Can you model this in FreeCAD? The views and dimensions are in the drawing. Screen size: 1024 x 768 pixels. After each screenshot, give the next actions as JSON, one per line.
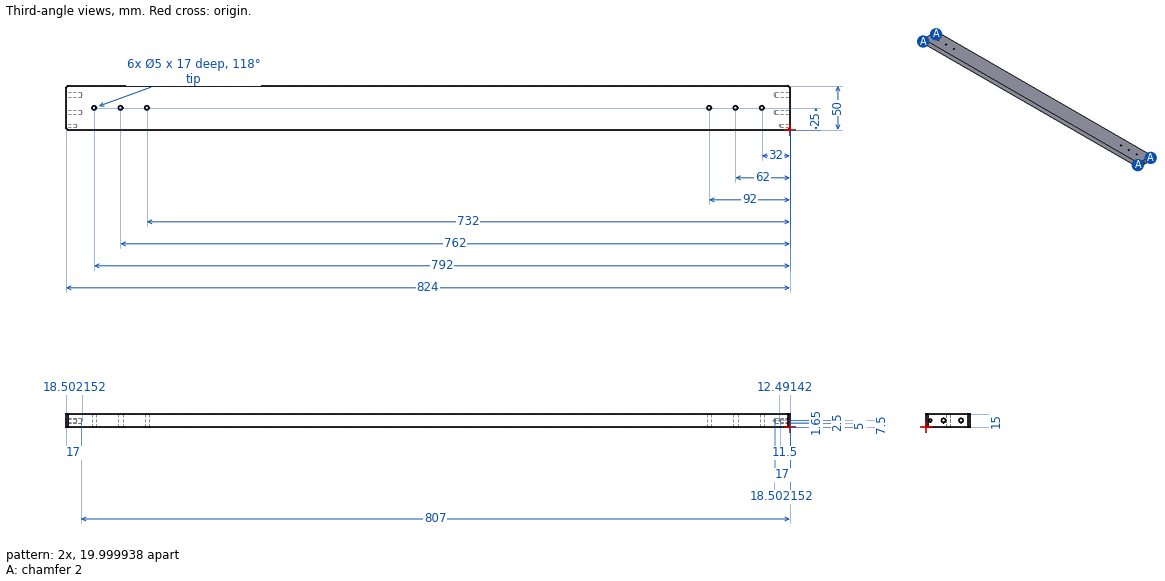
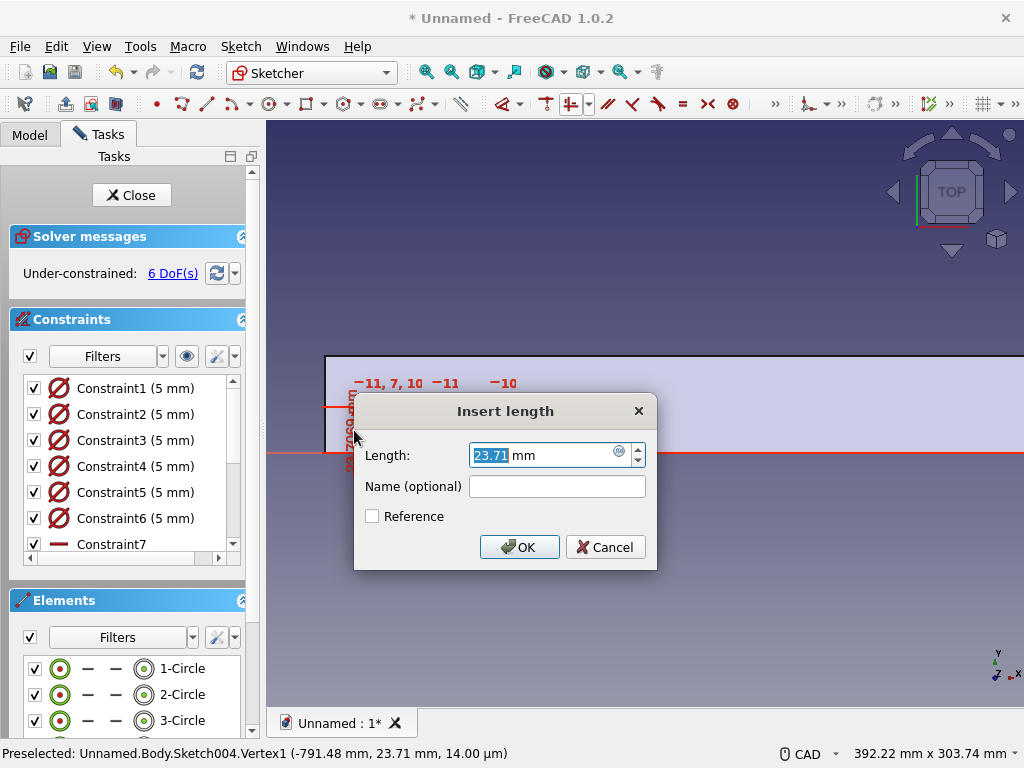
{"action": "type", "text": "25"}
{"action": "key", "text": "Return"}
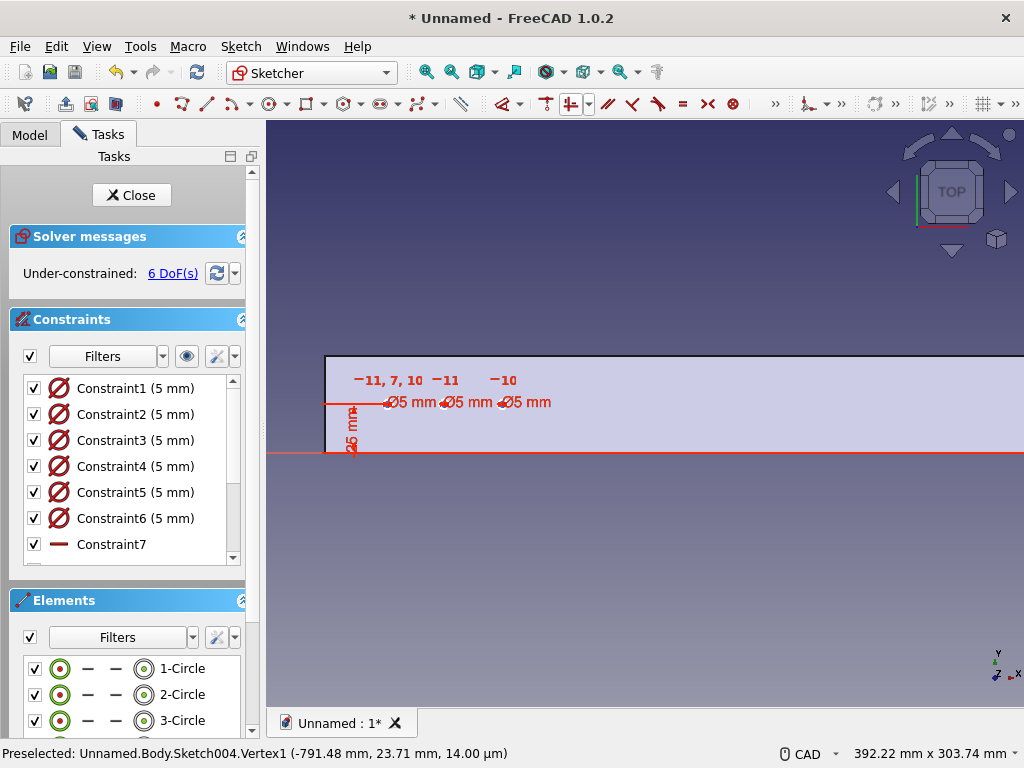
{"action": "scroll", "coordinate": [389, 409], "scroll_direction": "down", "scroll_amount": 7}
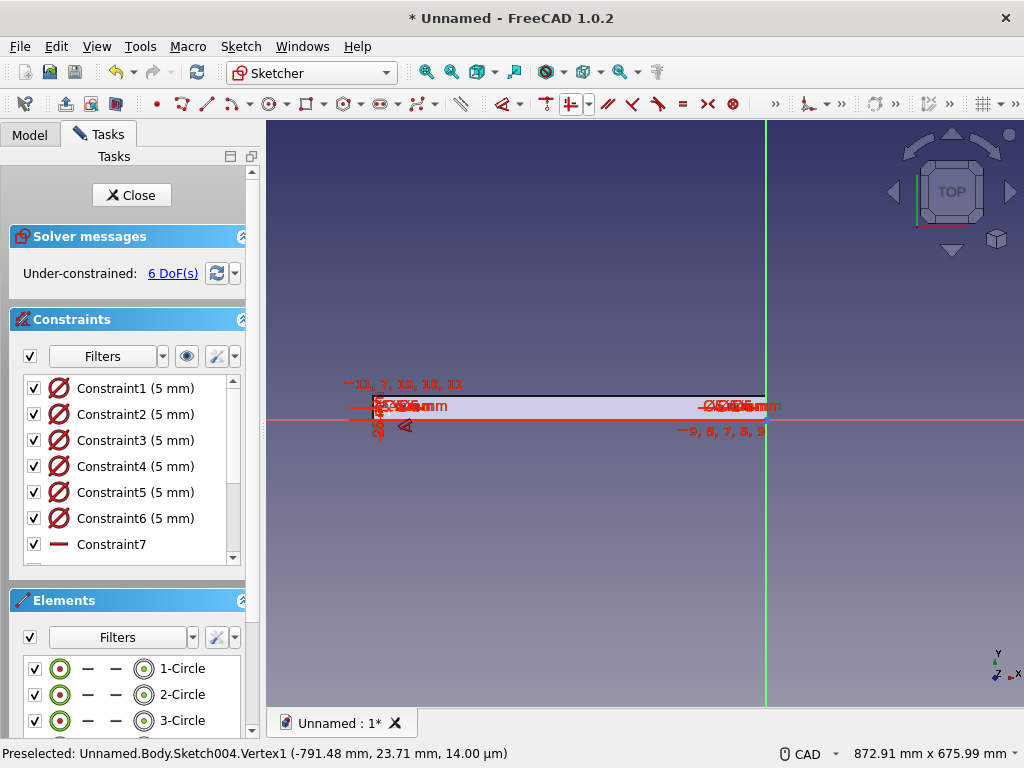
{"action": "scroll", "coordinate": [751, 408], "scroll_direction": "up", "scroll_amount": 5}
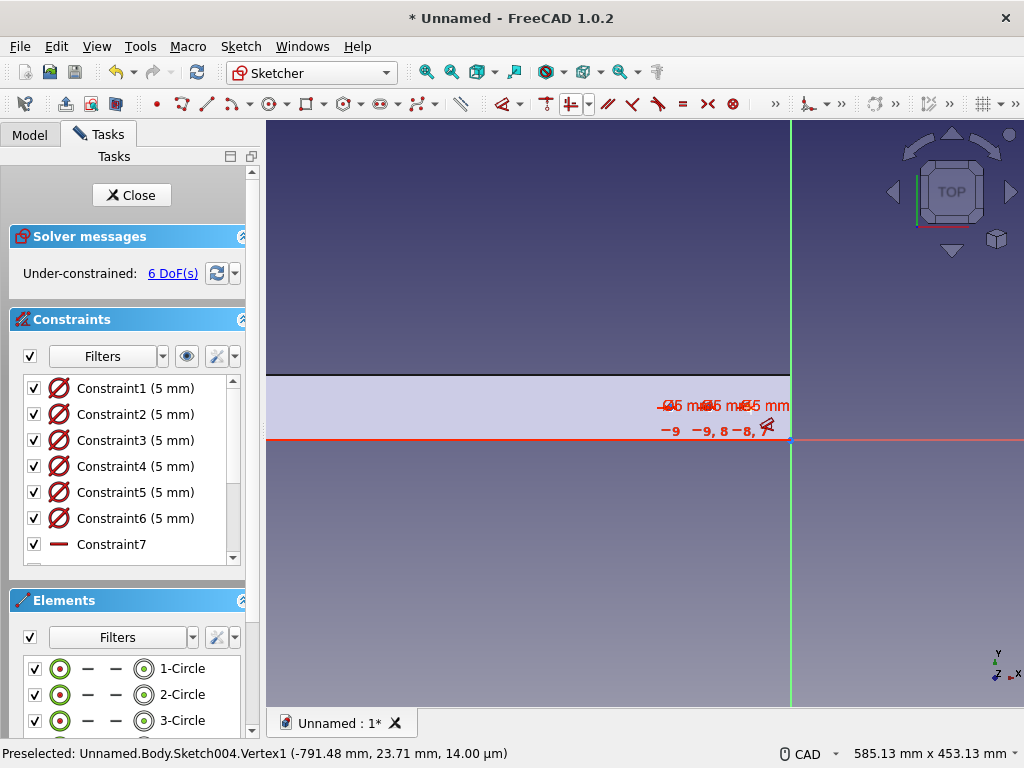
{"action": "left_click", "coordinate": [749, 408]}
{"action": "left_click", "coordinate": [770, 474]}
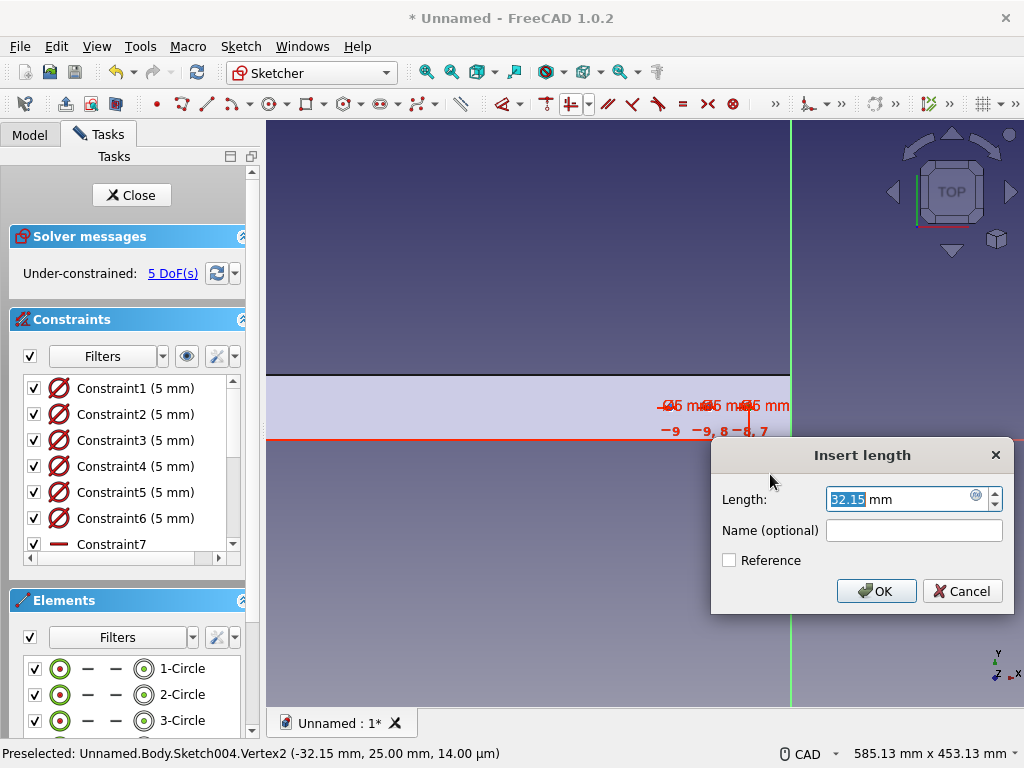
{"action": "type", "text": "32"}
{"action": "key", "text": "Return"}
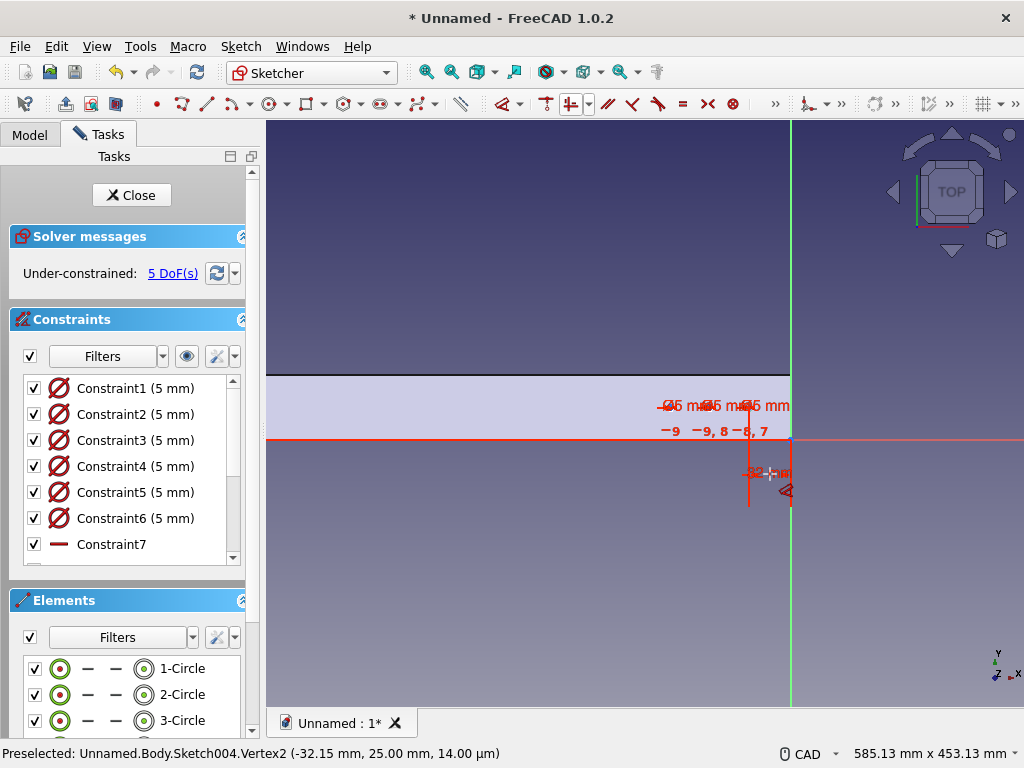
{"action": "left_click", "coordinate": [710, 408]}
{"action": "left_click", "coordinate": [750, 374]}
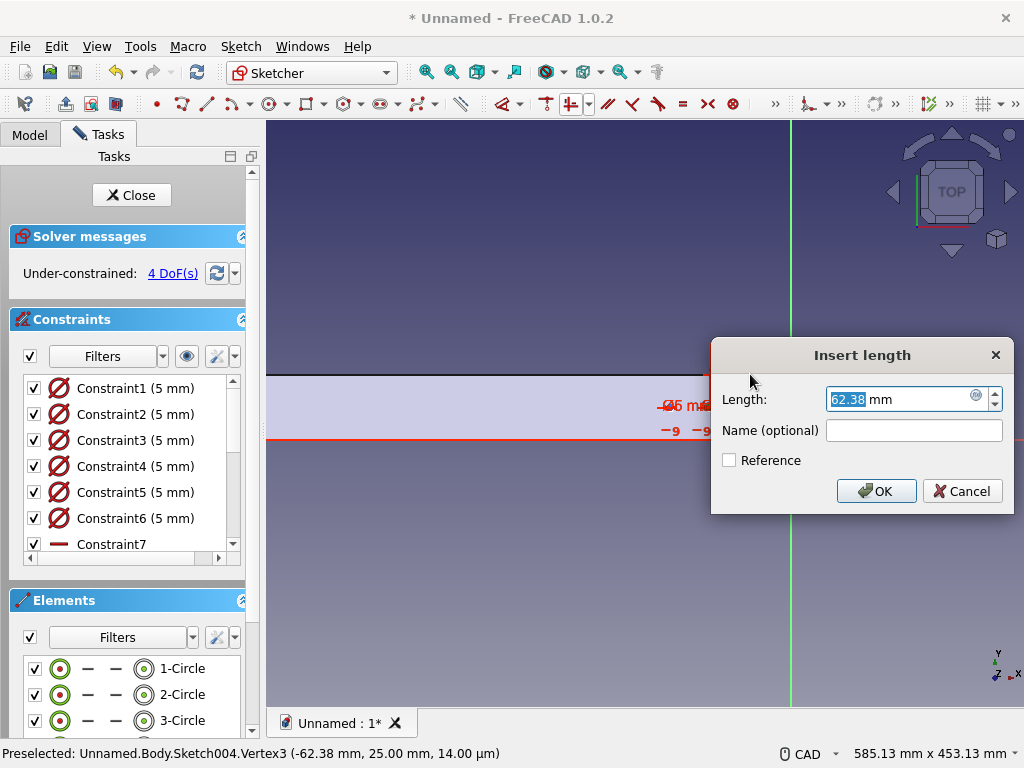
{"action": "type", "text": "62"}
{"action": "key", "text": "Return"}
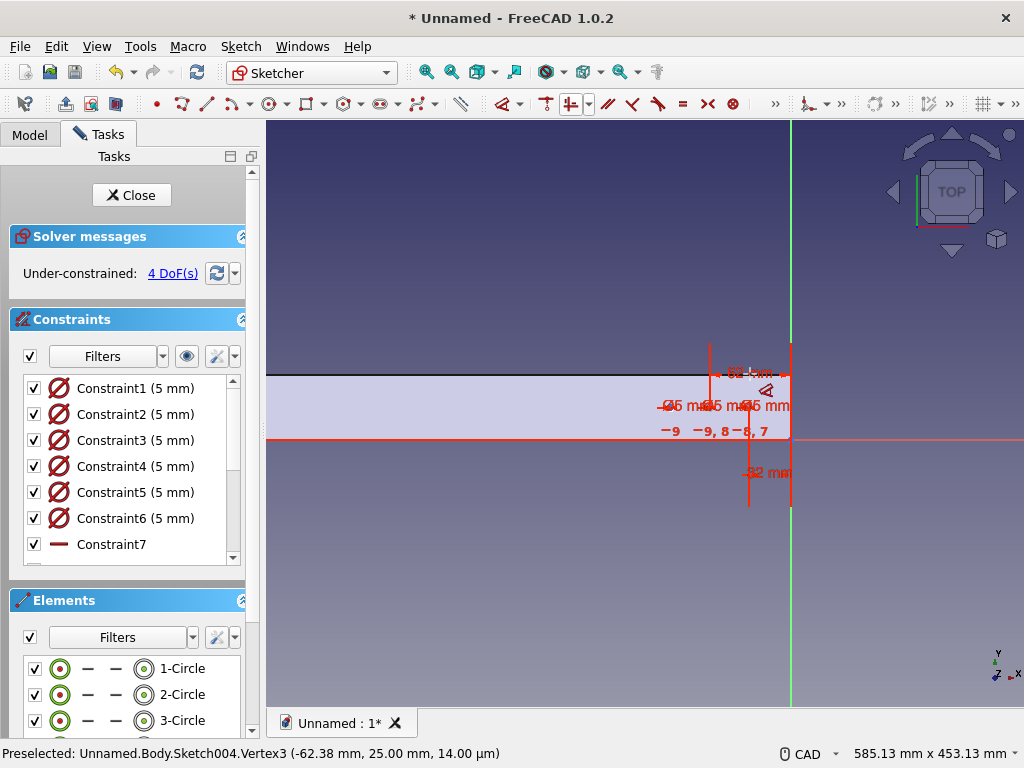
{"action": "left_click", "coordinate": [671, 408]}
{"action": "left_click", "coordinate": [689, 474]}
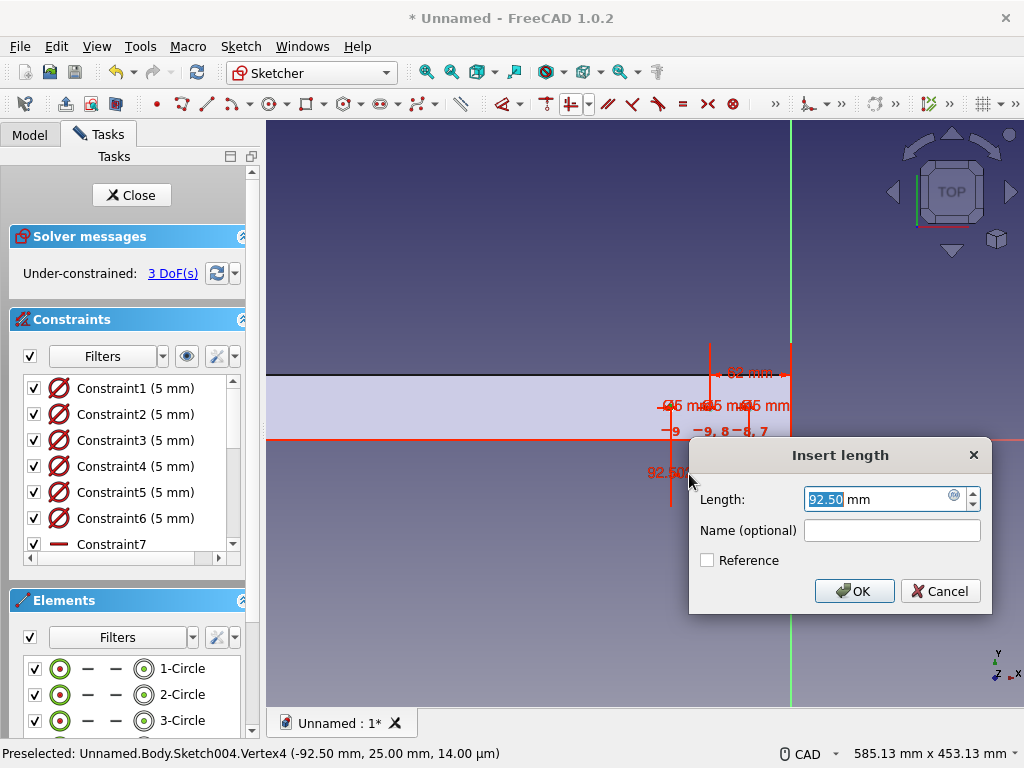
{"action": "type", "text": "92"}
{"action": "key", "text": "Return"}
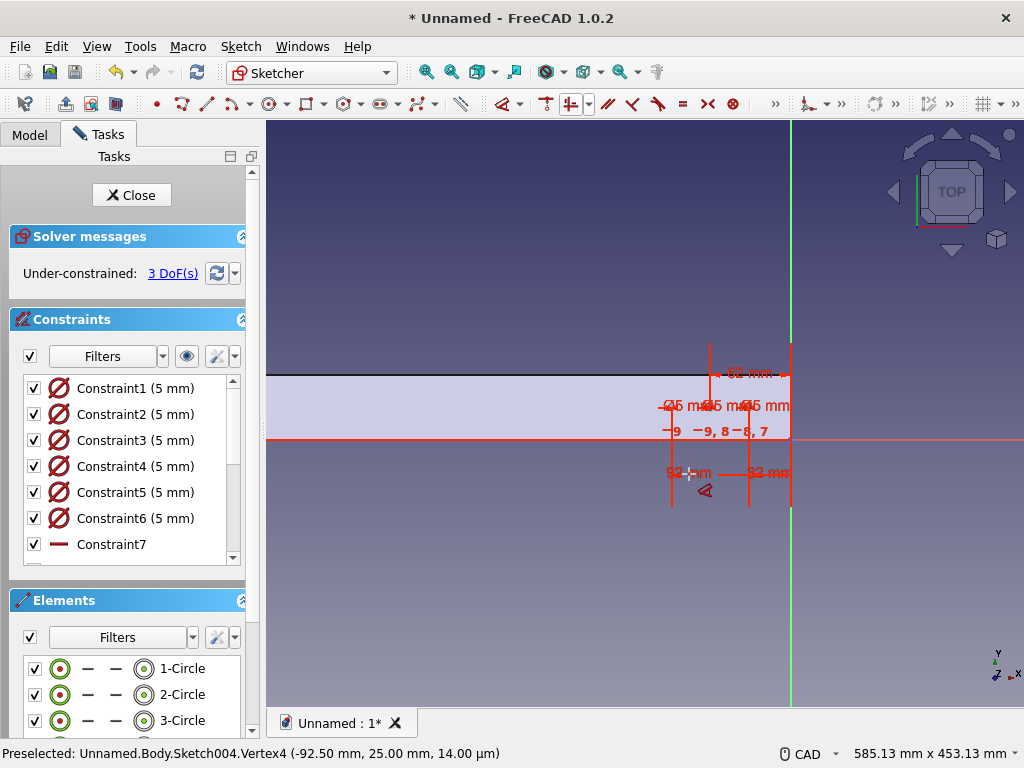
{"action": "scroll", "coordinate": [751, 408], "scroll_direction": "down", "scroll_amount": 5}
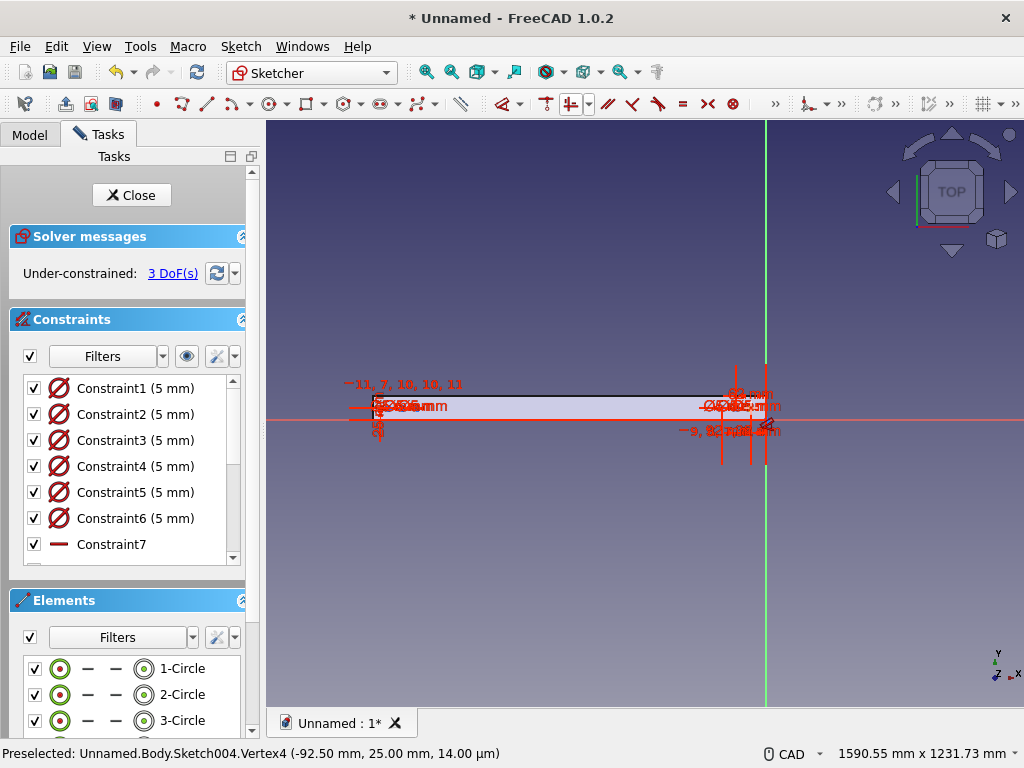
{"action": "left_click", "coordinate": [389, 408]}
{"action": "left_click", "coordinate": [577, 454]}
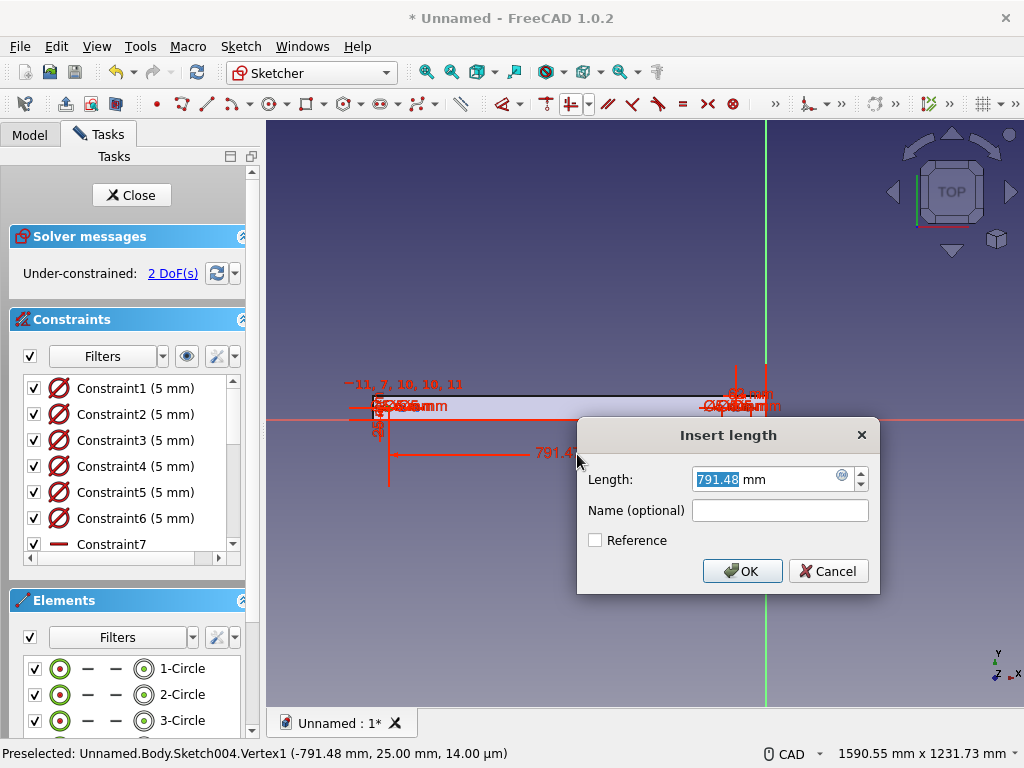
{"action": "type", "text": "792"}
{"action": "key", "text": "Return"}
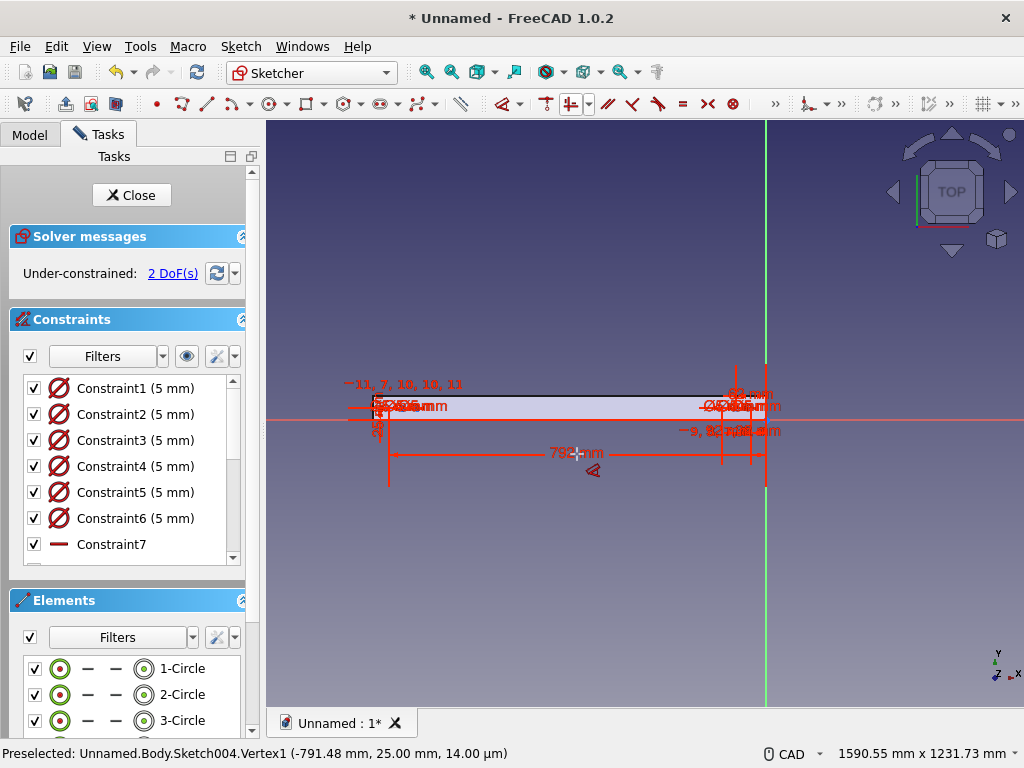
{"action": "left_click", "coordinate": [417, 408]}
{"action": "left_click", "coordinate": [672, 454]}